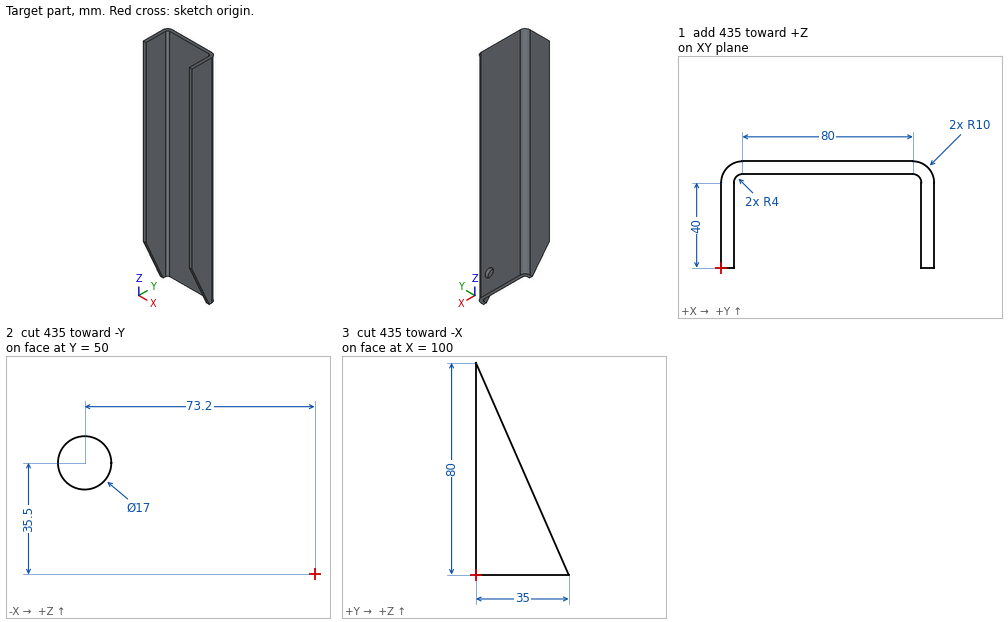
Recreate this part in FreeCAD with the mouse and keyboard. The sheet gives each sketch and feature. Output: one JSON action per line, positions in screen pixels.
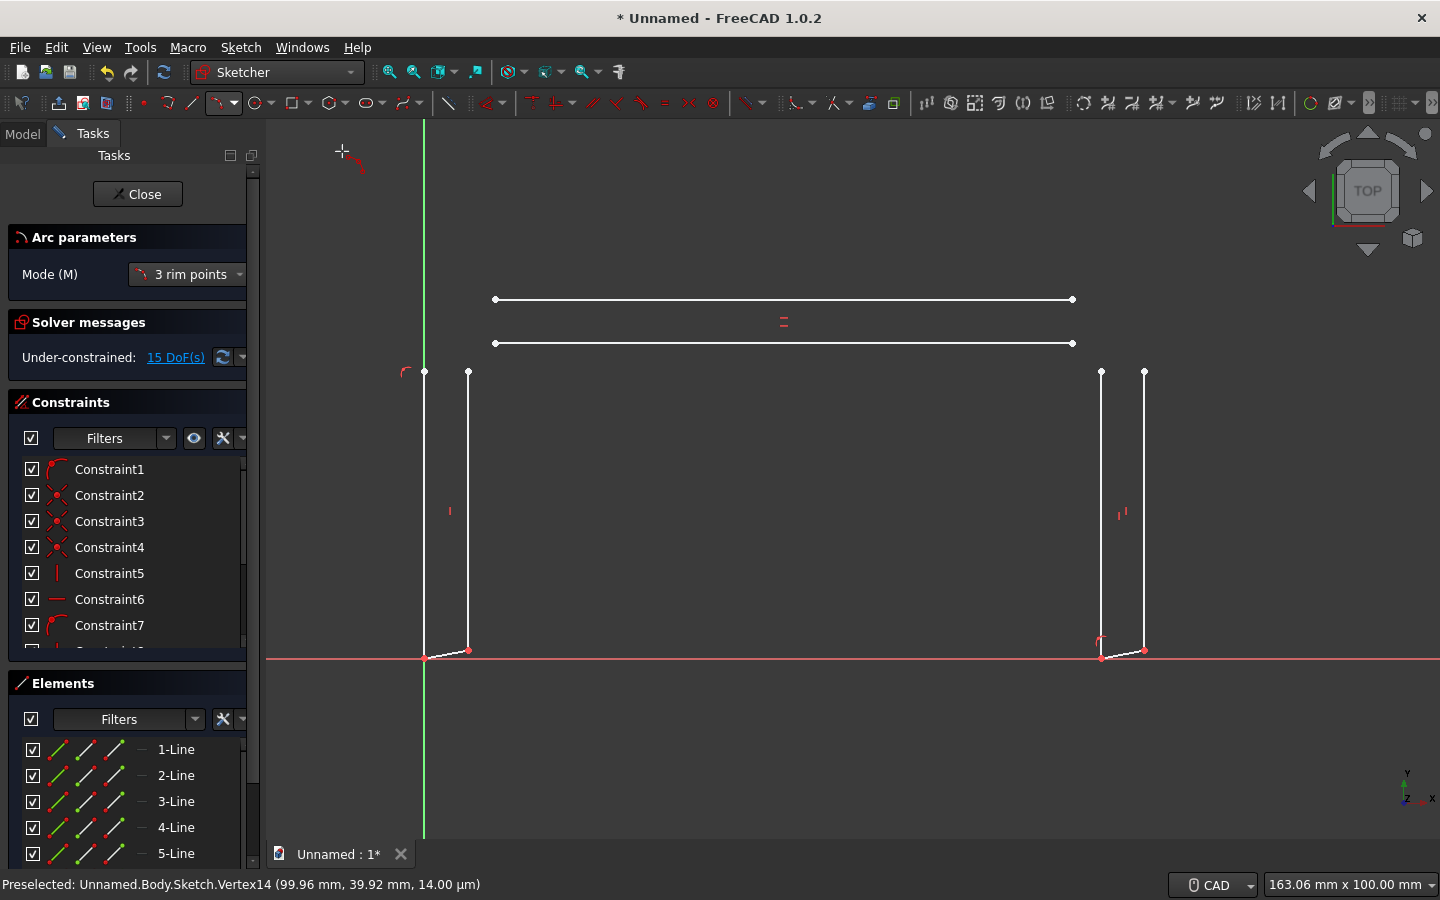
{"action": "left_click", "coordinate": [468, 371]}
{"action": "left_click", "coordinate": [496, 343]}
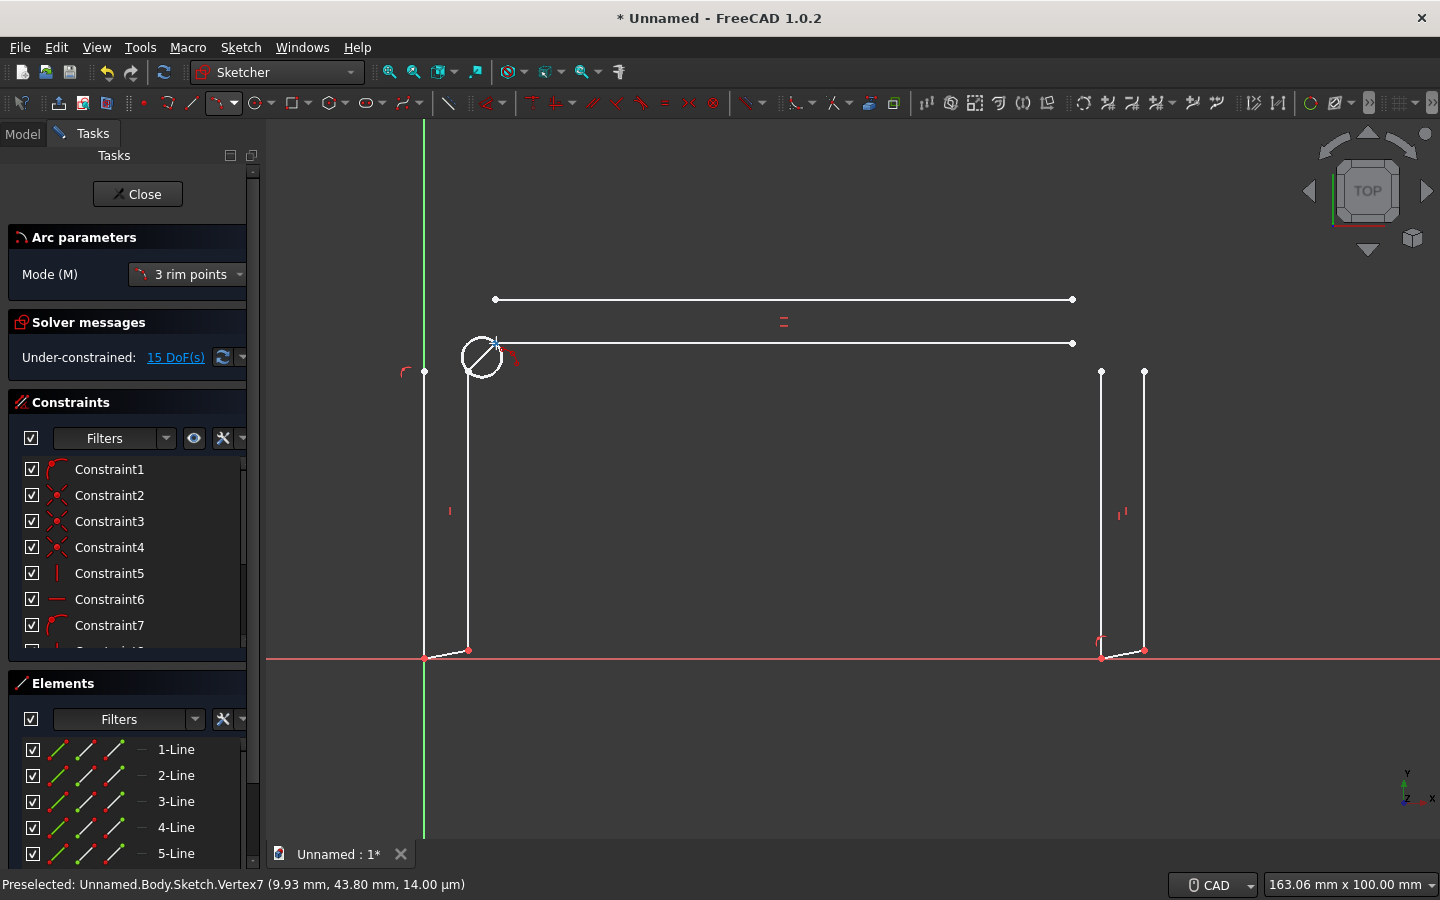
{"action": "scroll", "coordinate": [476, 350], "scroll_direction": "up", "scroll_amount": 4}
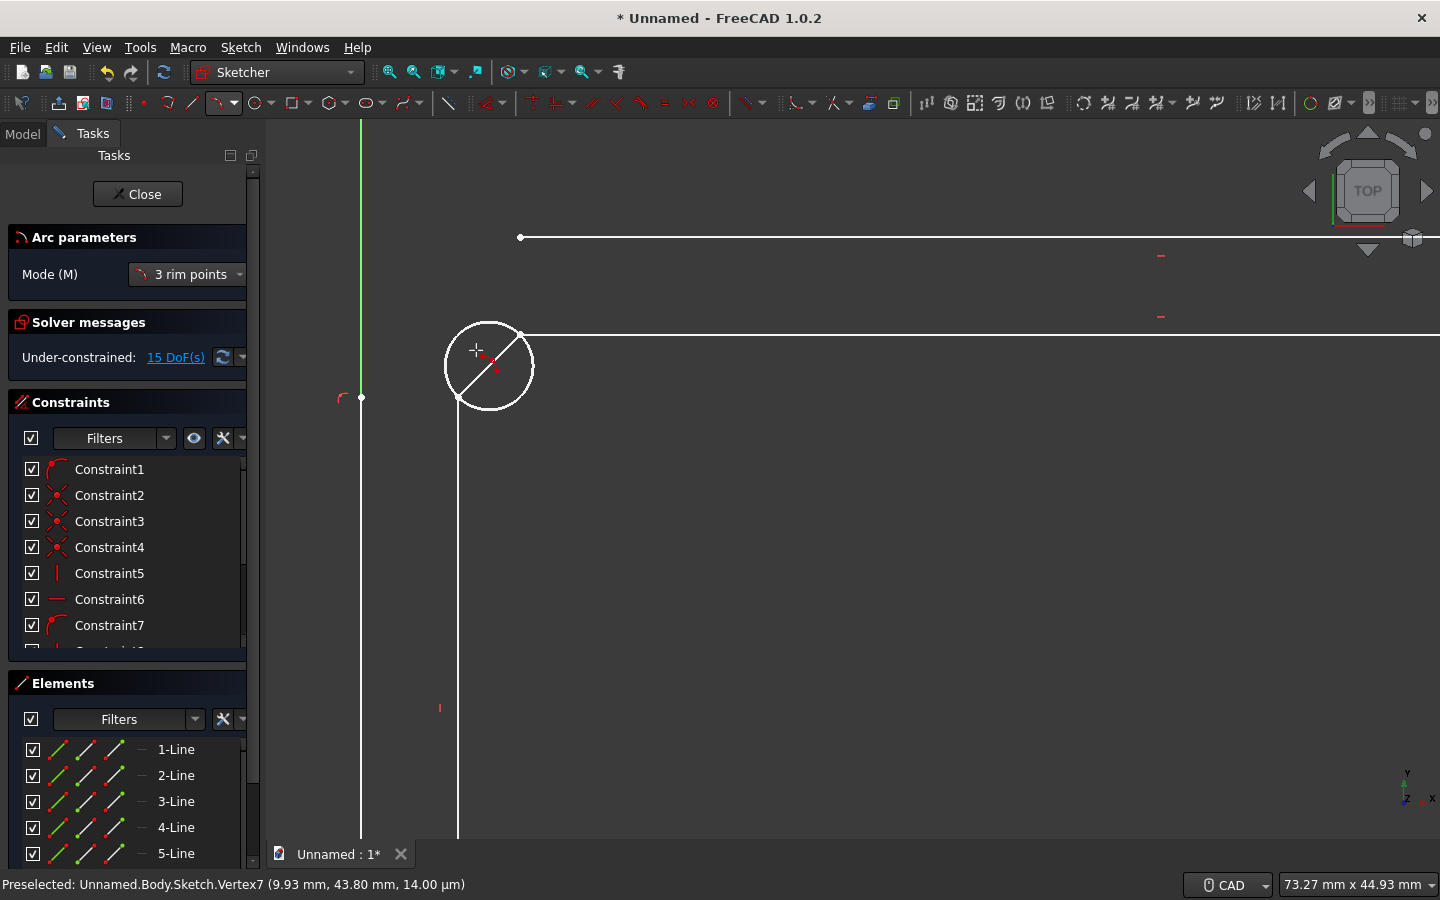
{"action": "left_click", "coordinate": [476, 350]}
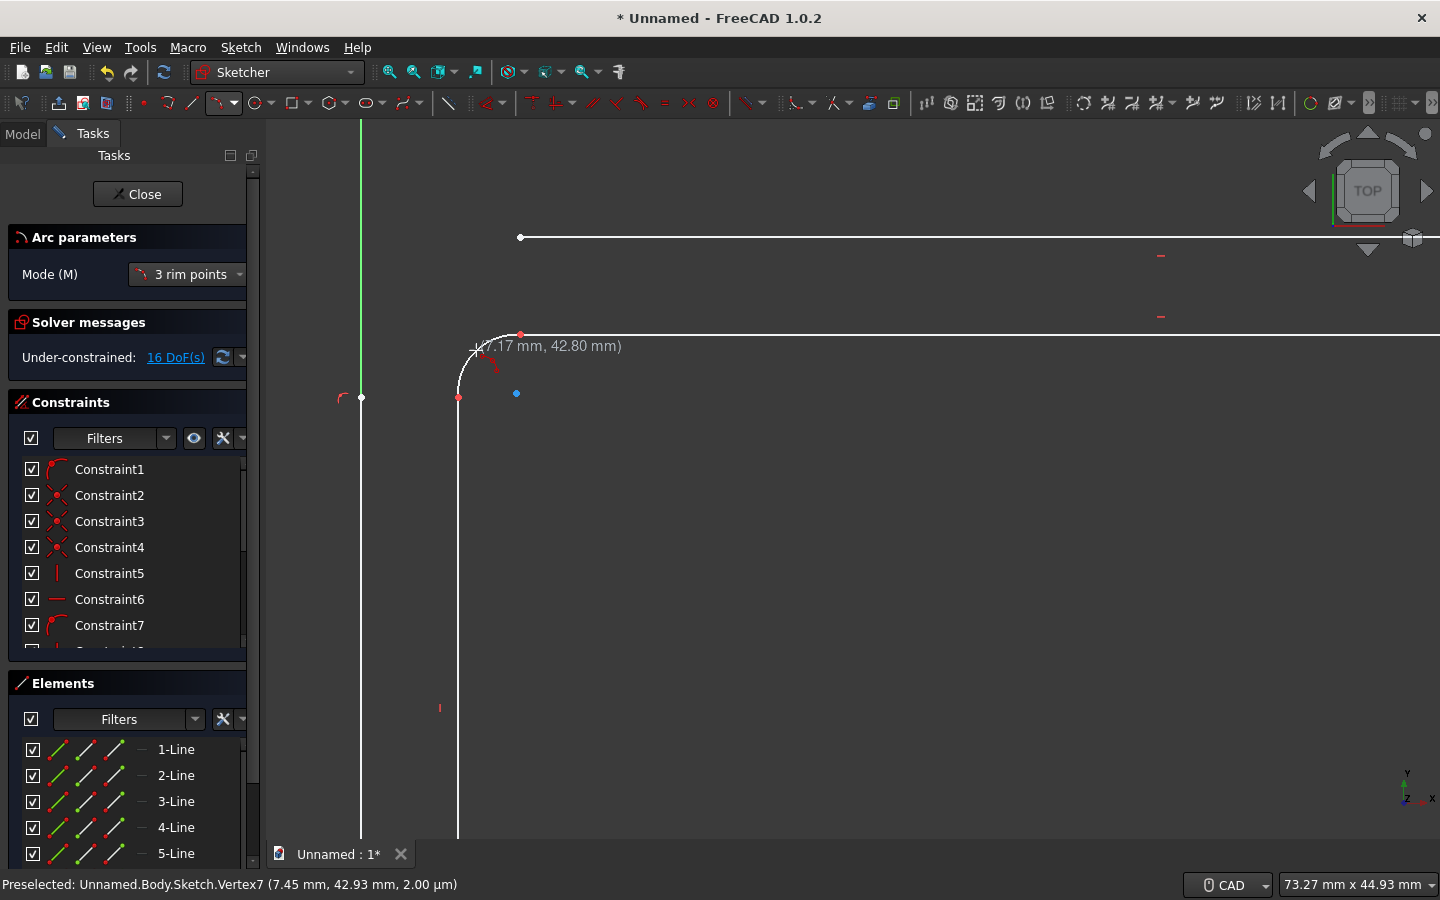
{"action": "scroll", "coordinate": [476, 351], "scroll_direction": "down", "scroll_amount": 4}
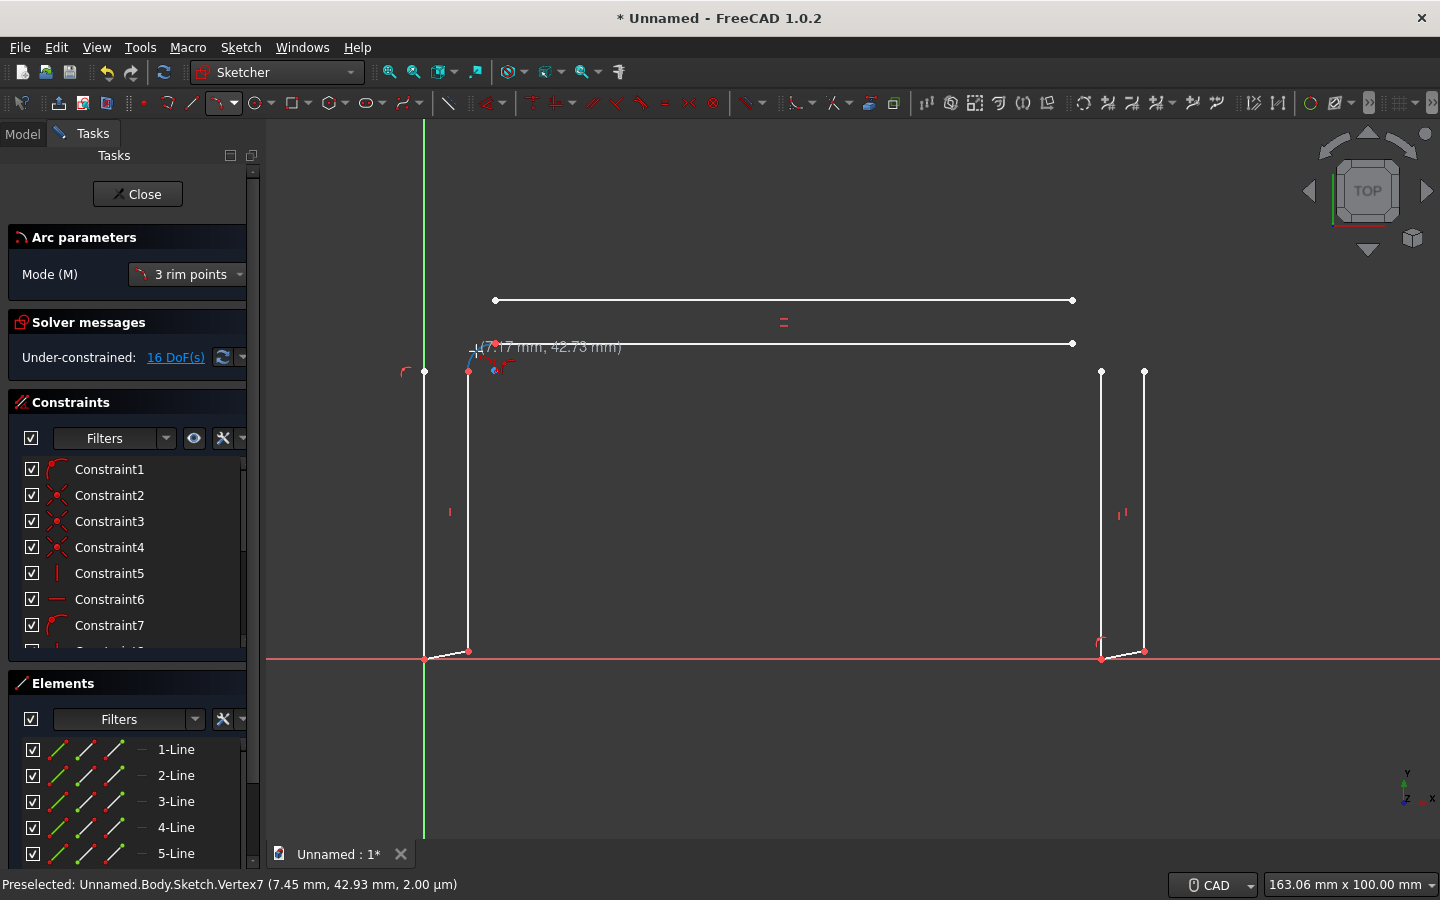
{"action": "left_click", "coordinate": [1072, 344]}
{"action": "left_click", "coordinate": [1101, 372]}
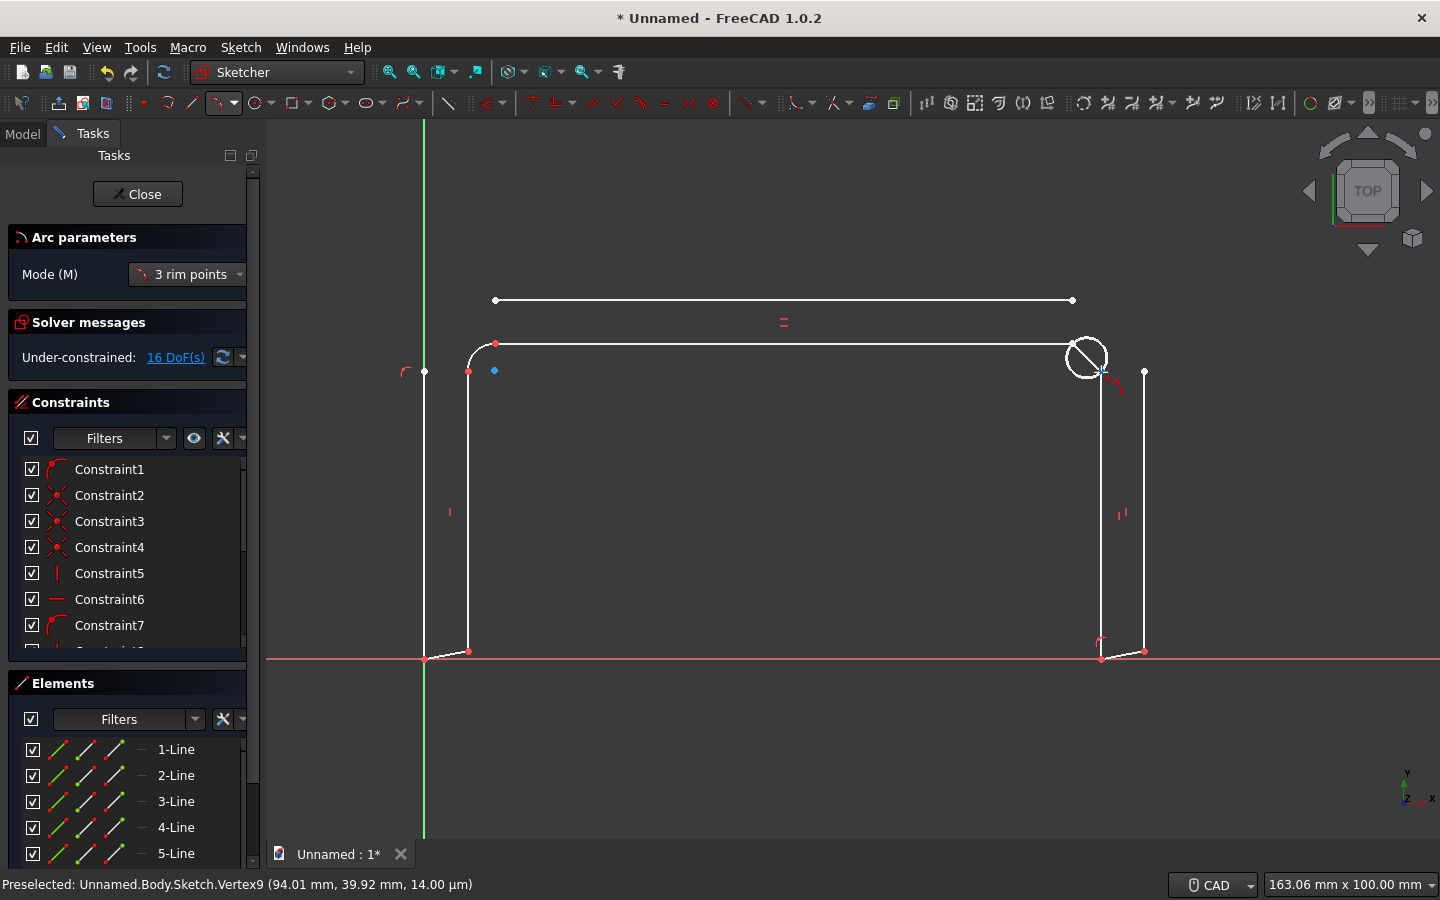
{"action": "scroll", "coordinate": [1093, 351], "scroll_direction": "up", "scroll_amount": 4}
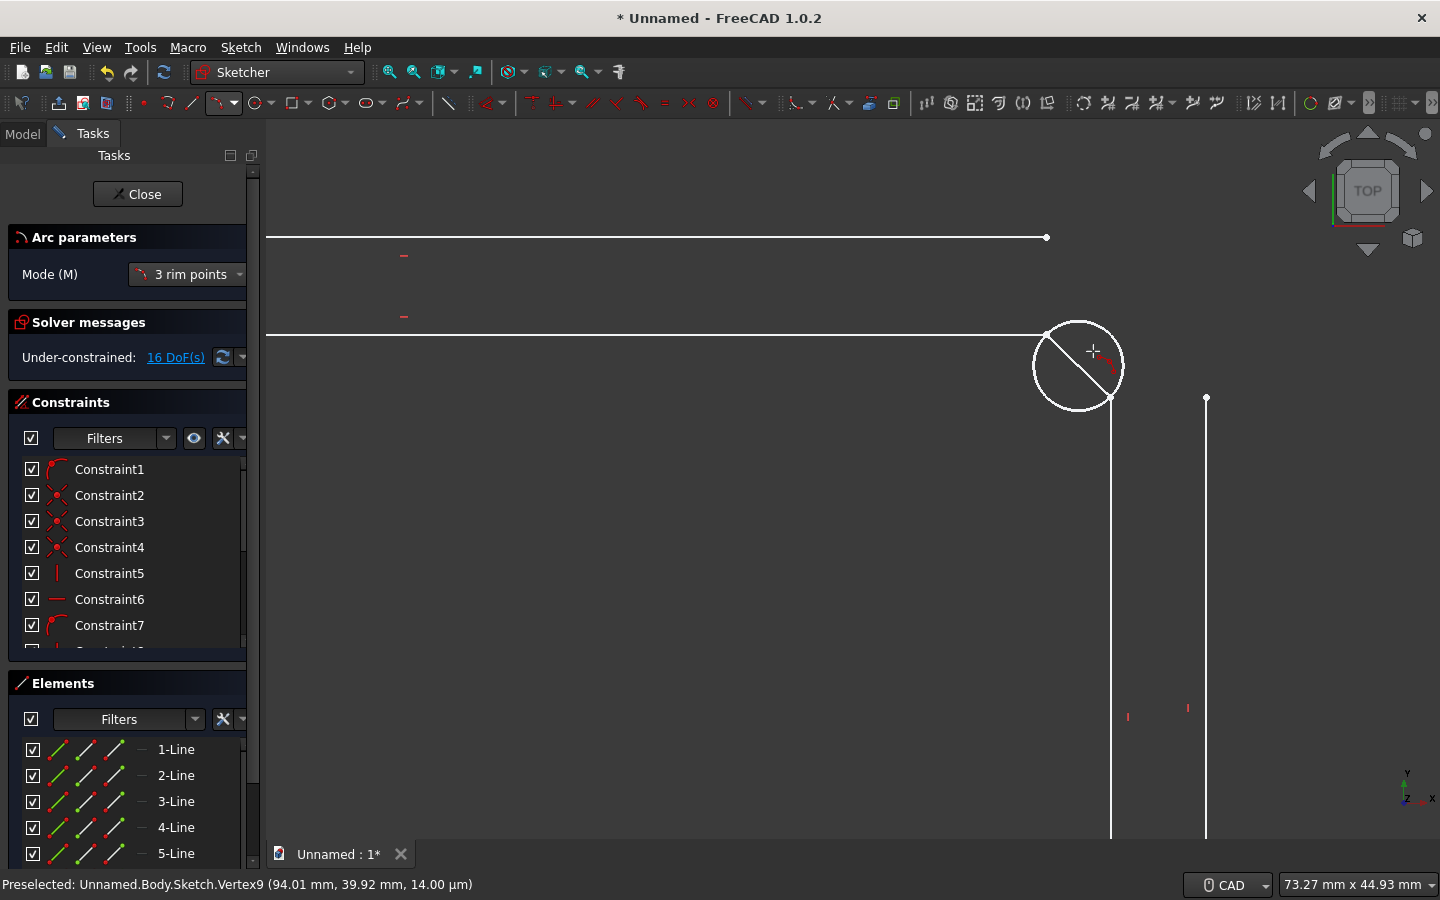
{"action": "left_click", "coordinate": [1092, 350]}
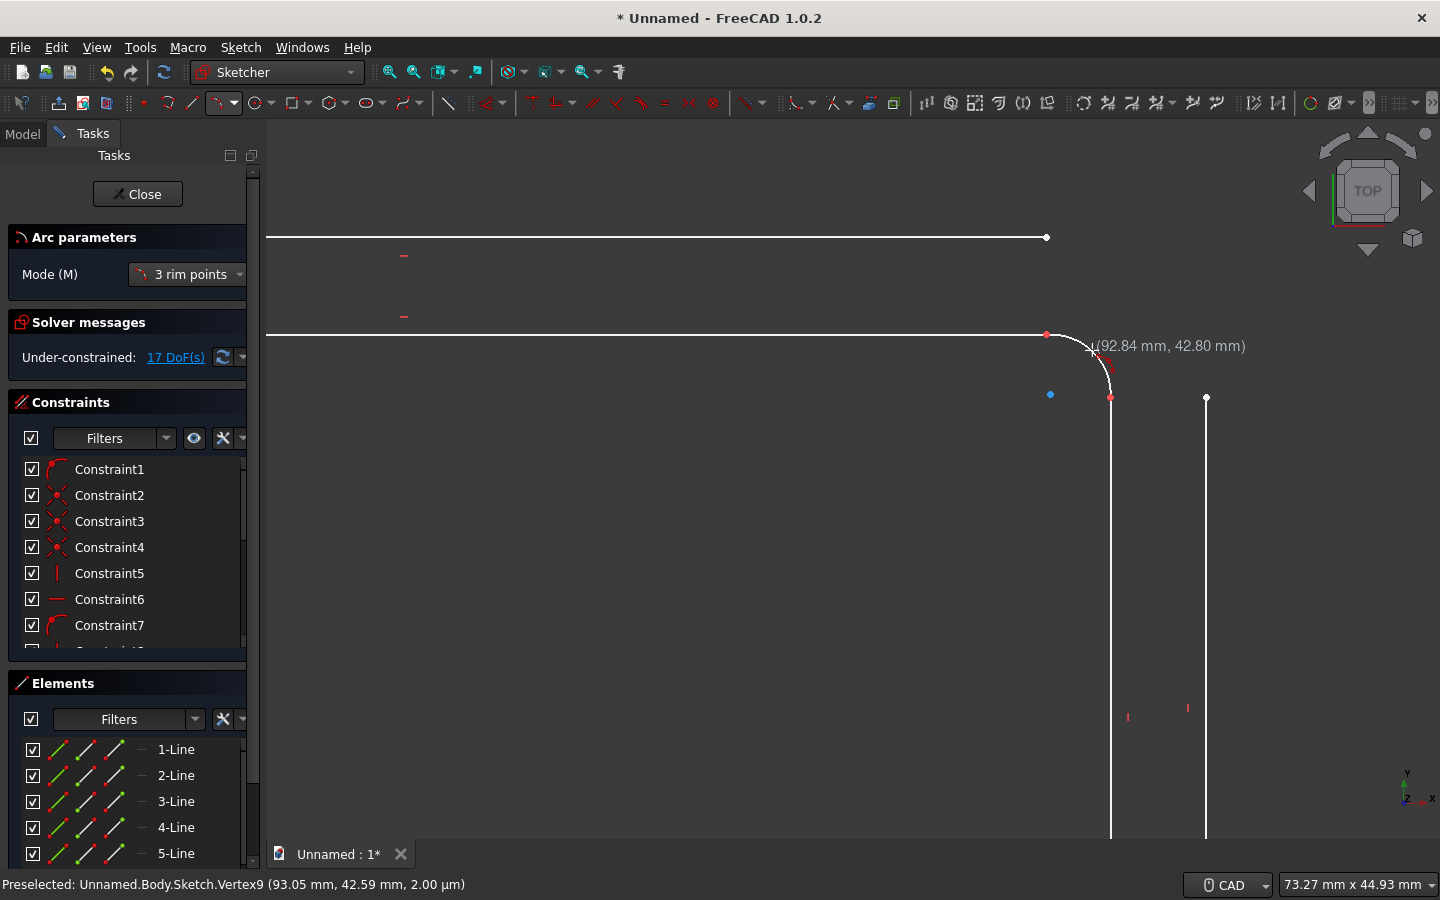
{"action": "left_click", "coordinate": [1206, 397]}
{"action": "left_click", "coordinate": [1046, 237]}
{"action": "left_click", "coordinate": [1160, 282]}